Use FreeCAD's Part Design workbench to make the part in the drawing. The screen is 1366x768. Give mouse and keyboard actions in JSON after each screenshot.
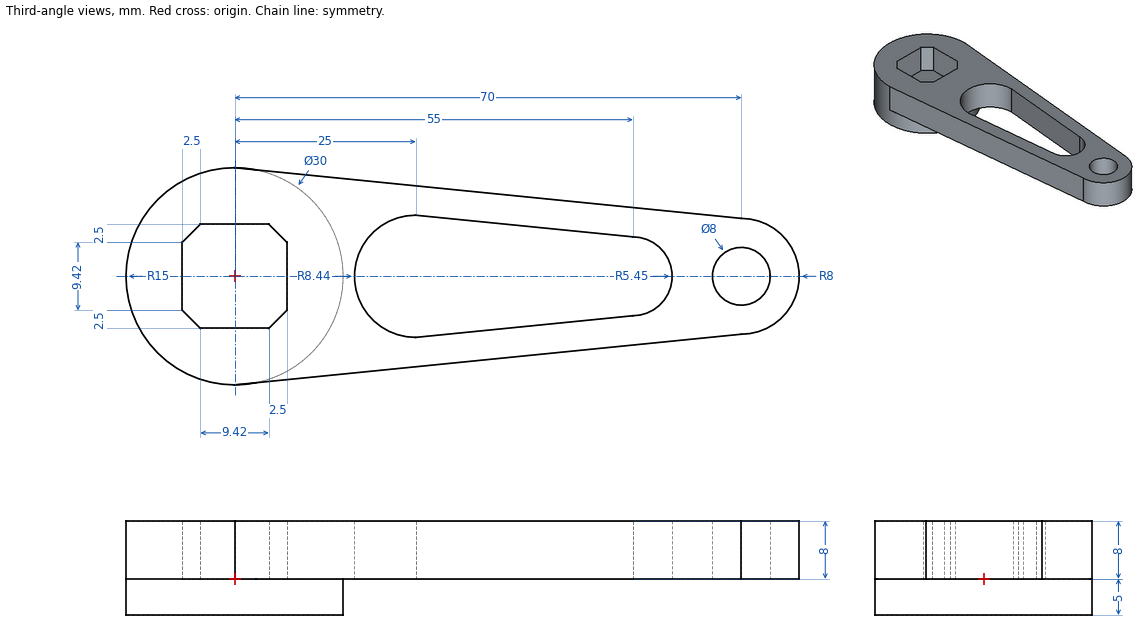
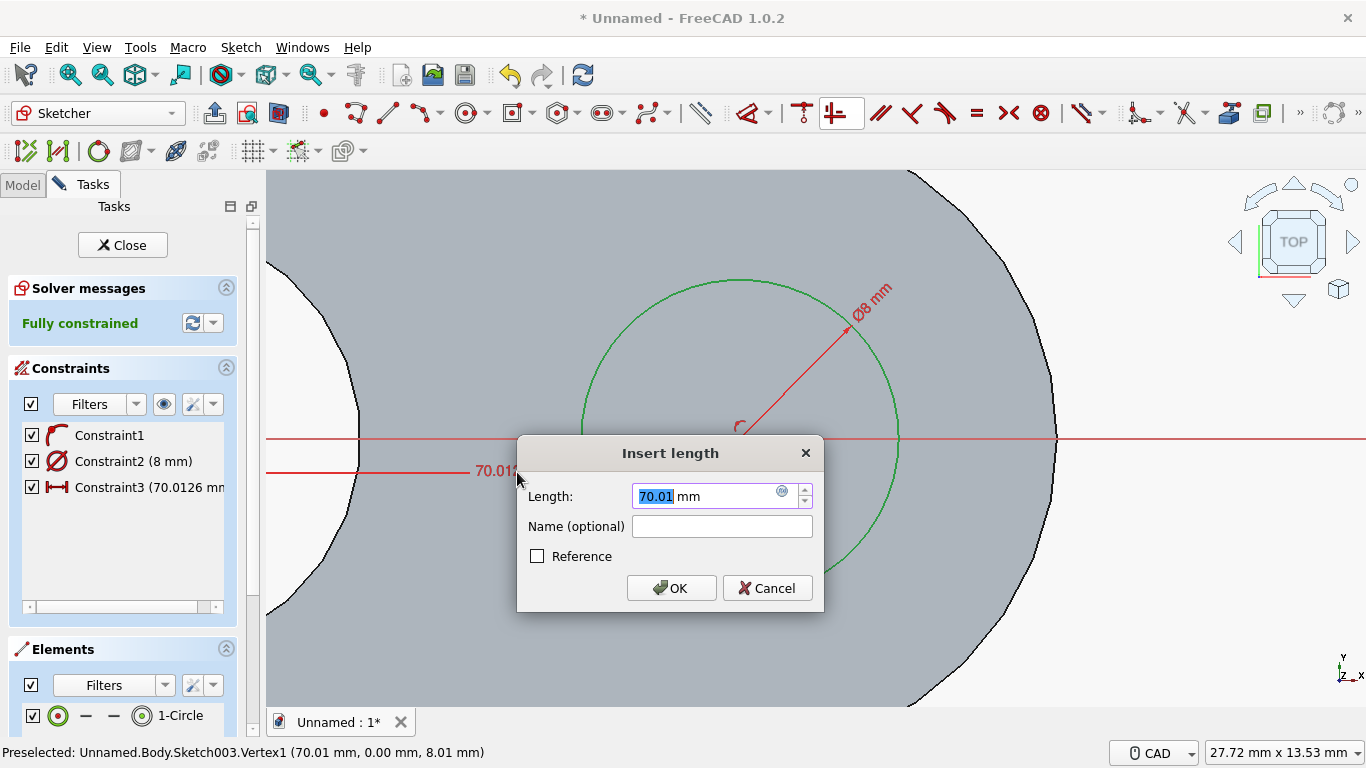
{"action": "type", "text": "70"}
{"action": "key", "text": "Return"}
{"action": "key", "text": "Escape"}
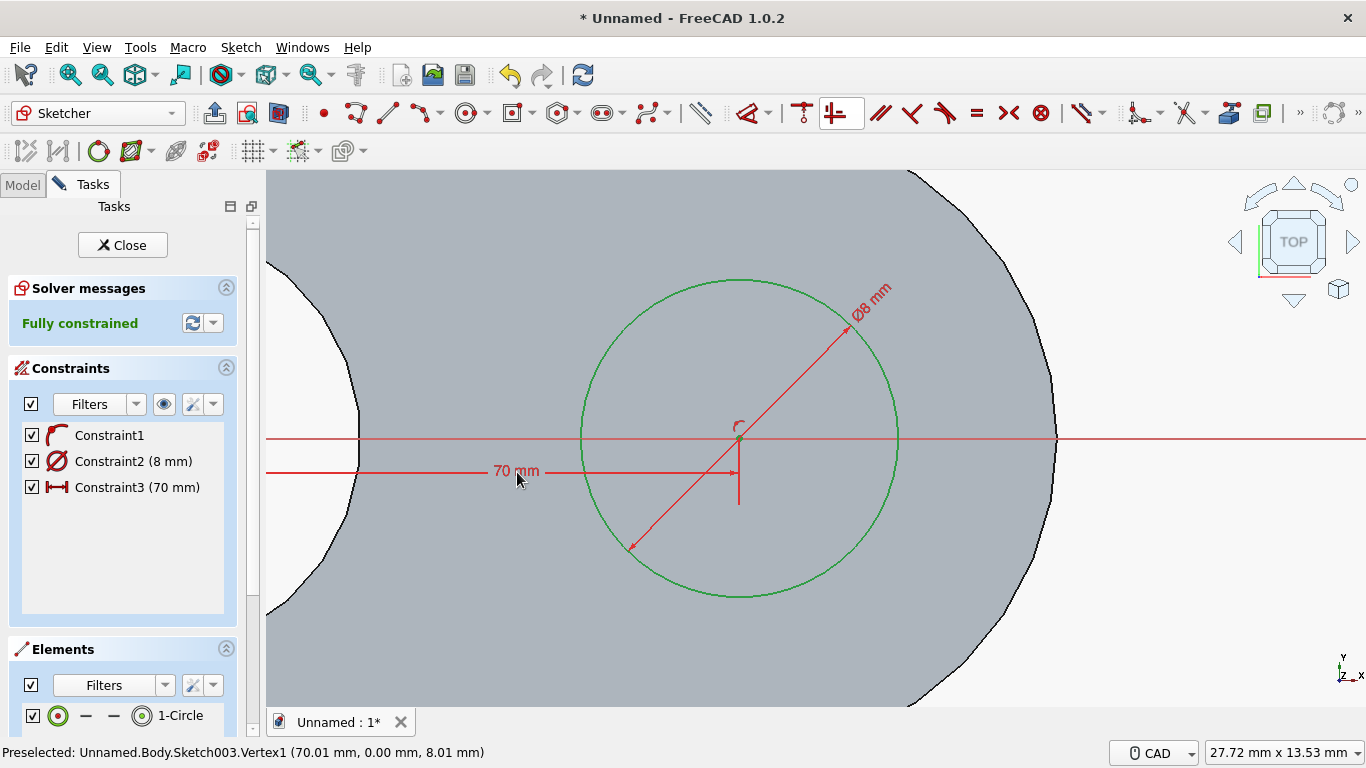
{"action": "left_click", "coordinate": [123, 245]}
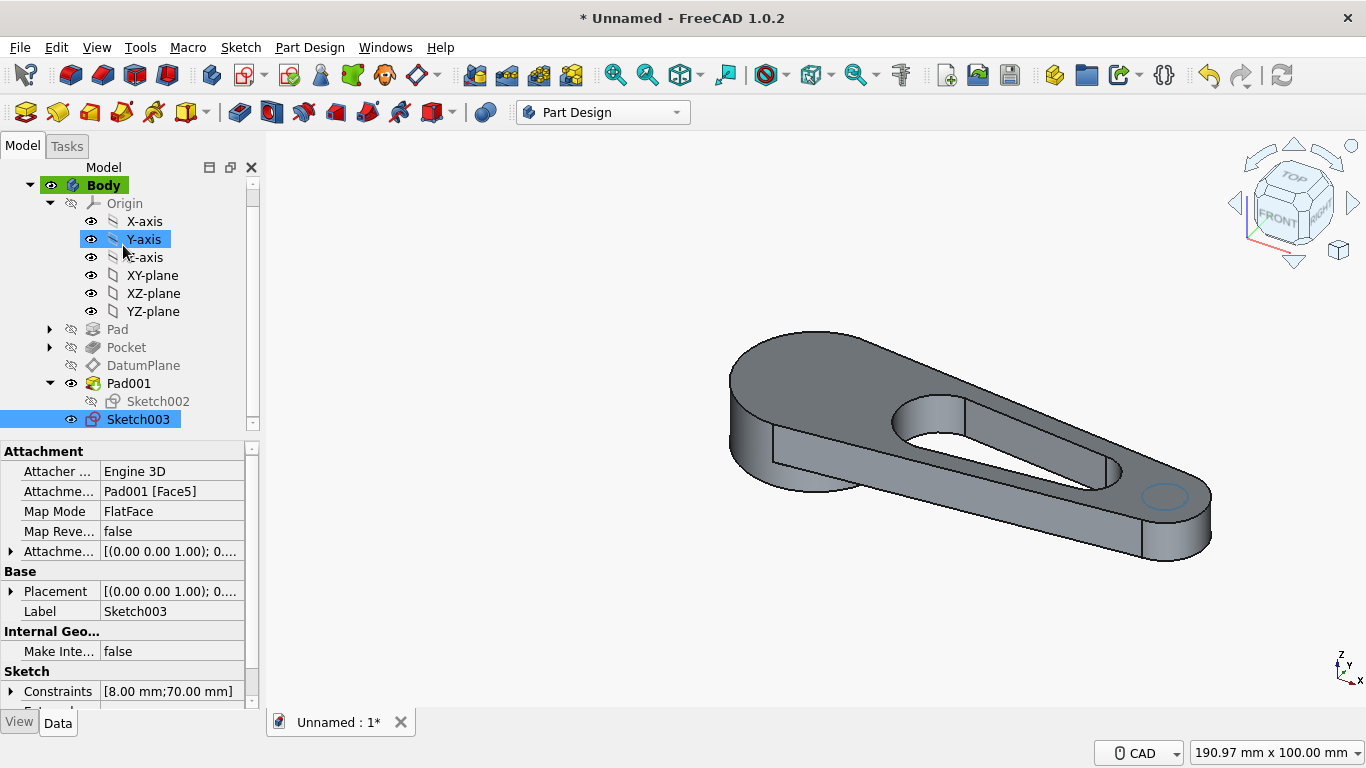
{"action": "left_click", "coordinate": [240, 112]}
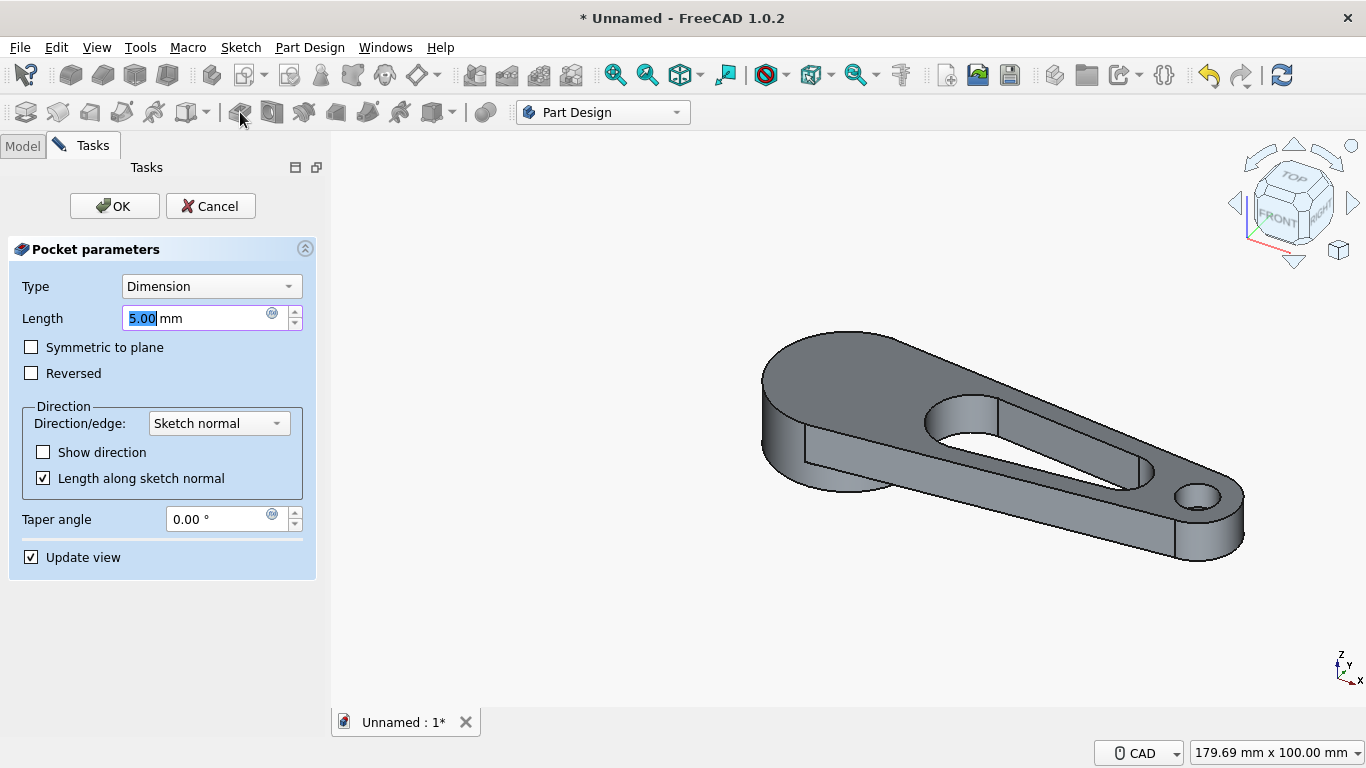
{"action": "type", "text": "8"}
{"action": "key", "text": "Tab"}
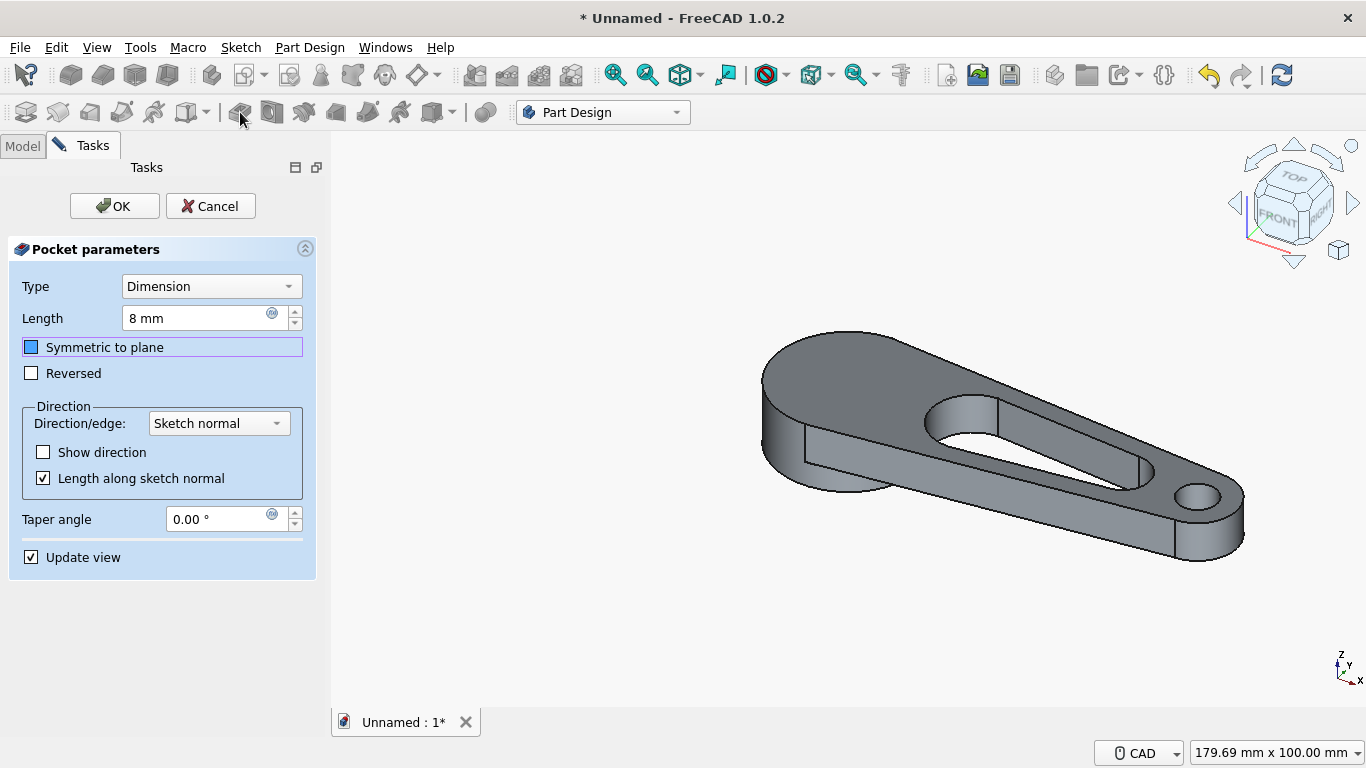
{"action": "left_click", "coordinate": [115, 206]}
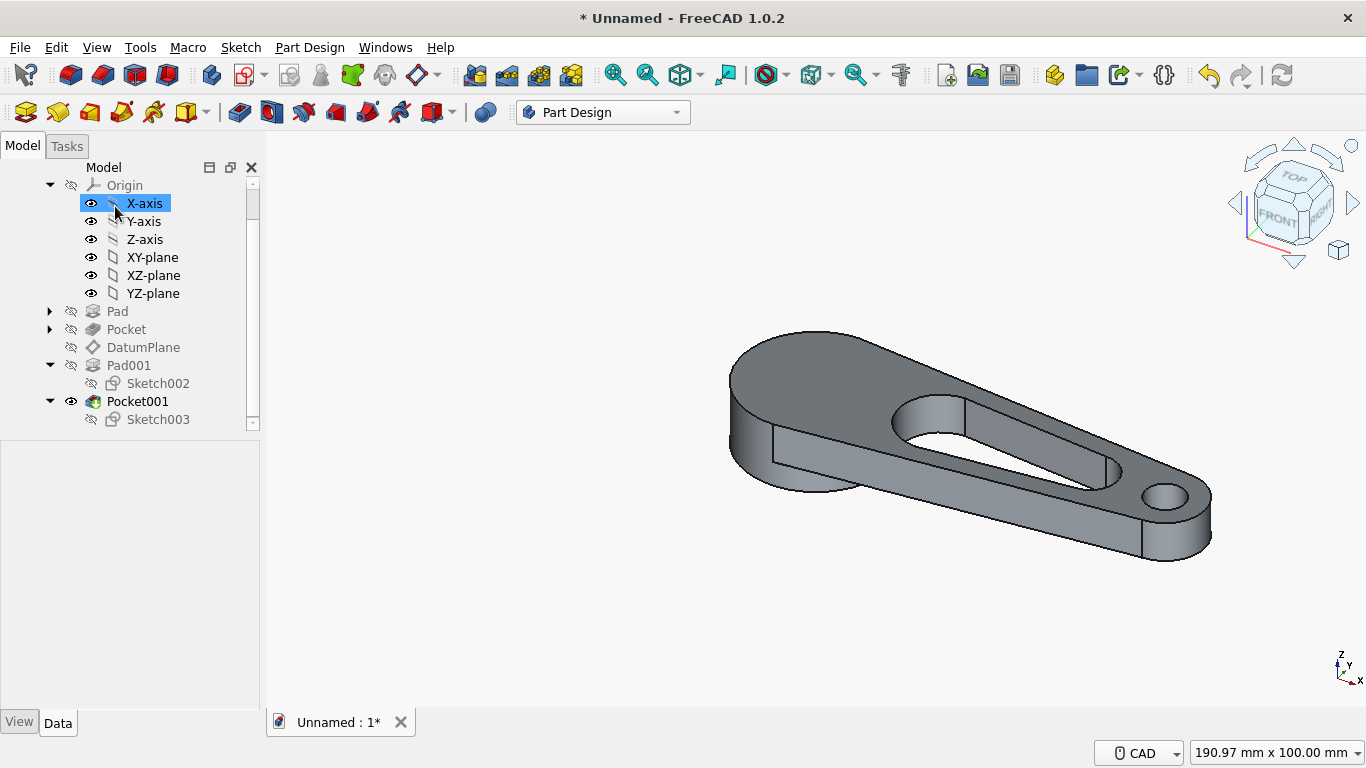
{"action": "left_click", "coordinate": [841, 388]}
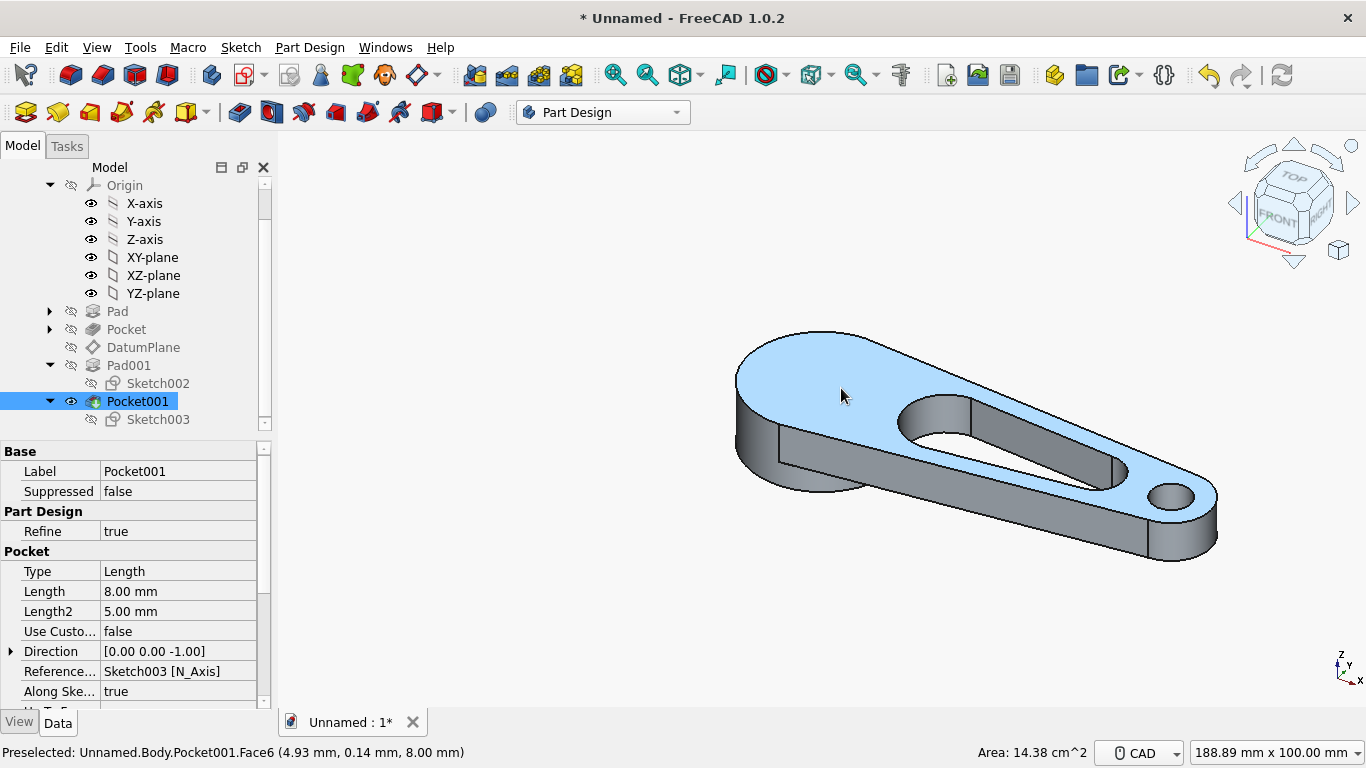
{"action": "left_click", "coordinate": [244, 76]}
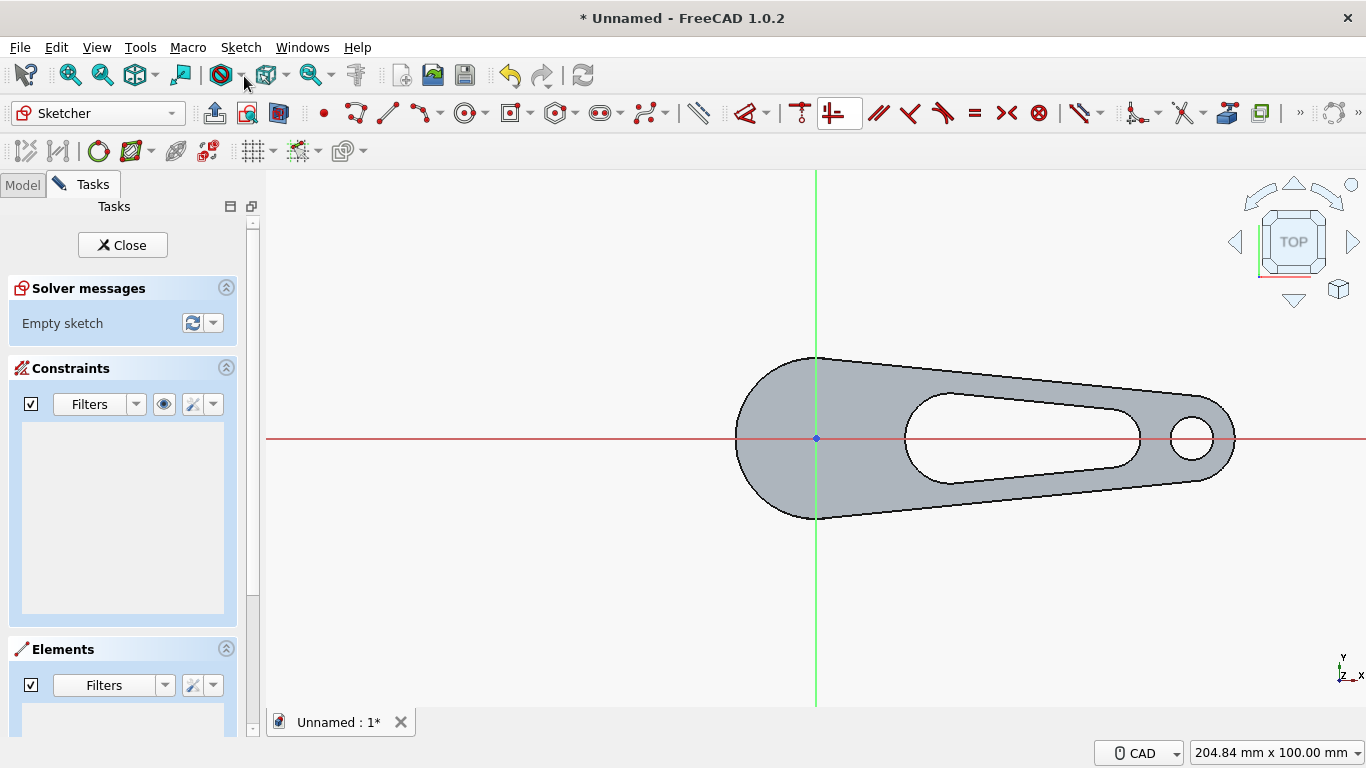
{"action": "scroll", "coordinate": [838, 438], "scroll_direction": "up", "scroll_amount": 7}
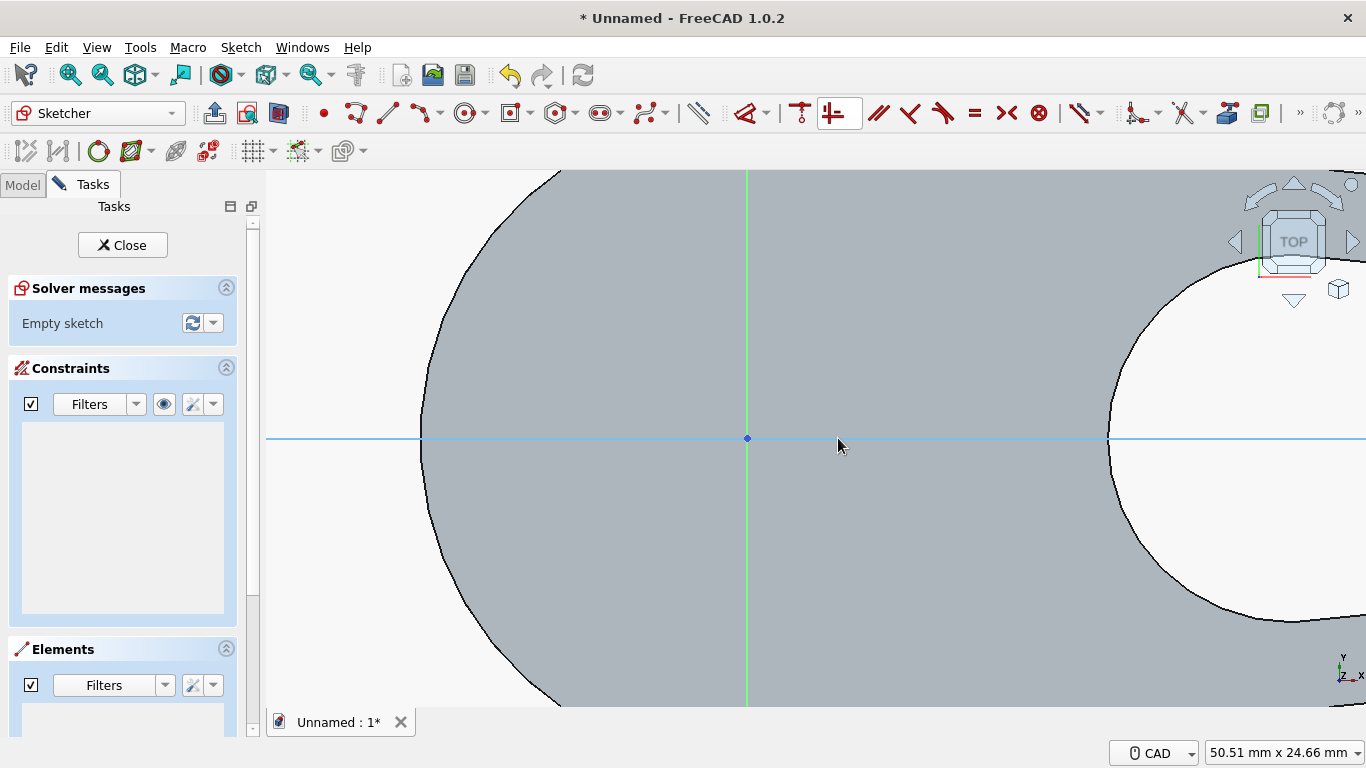
{"action": "key", "text": "g m"}